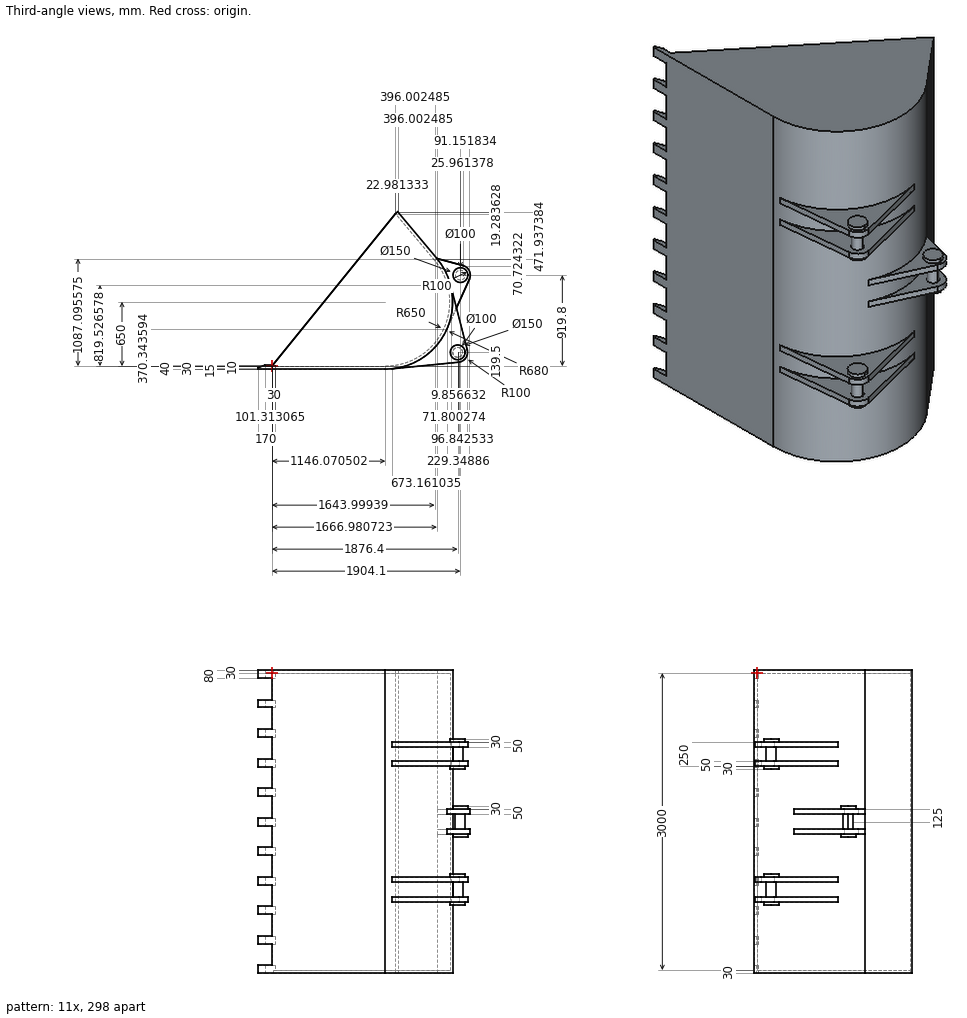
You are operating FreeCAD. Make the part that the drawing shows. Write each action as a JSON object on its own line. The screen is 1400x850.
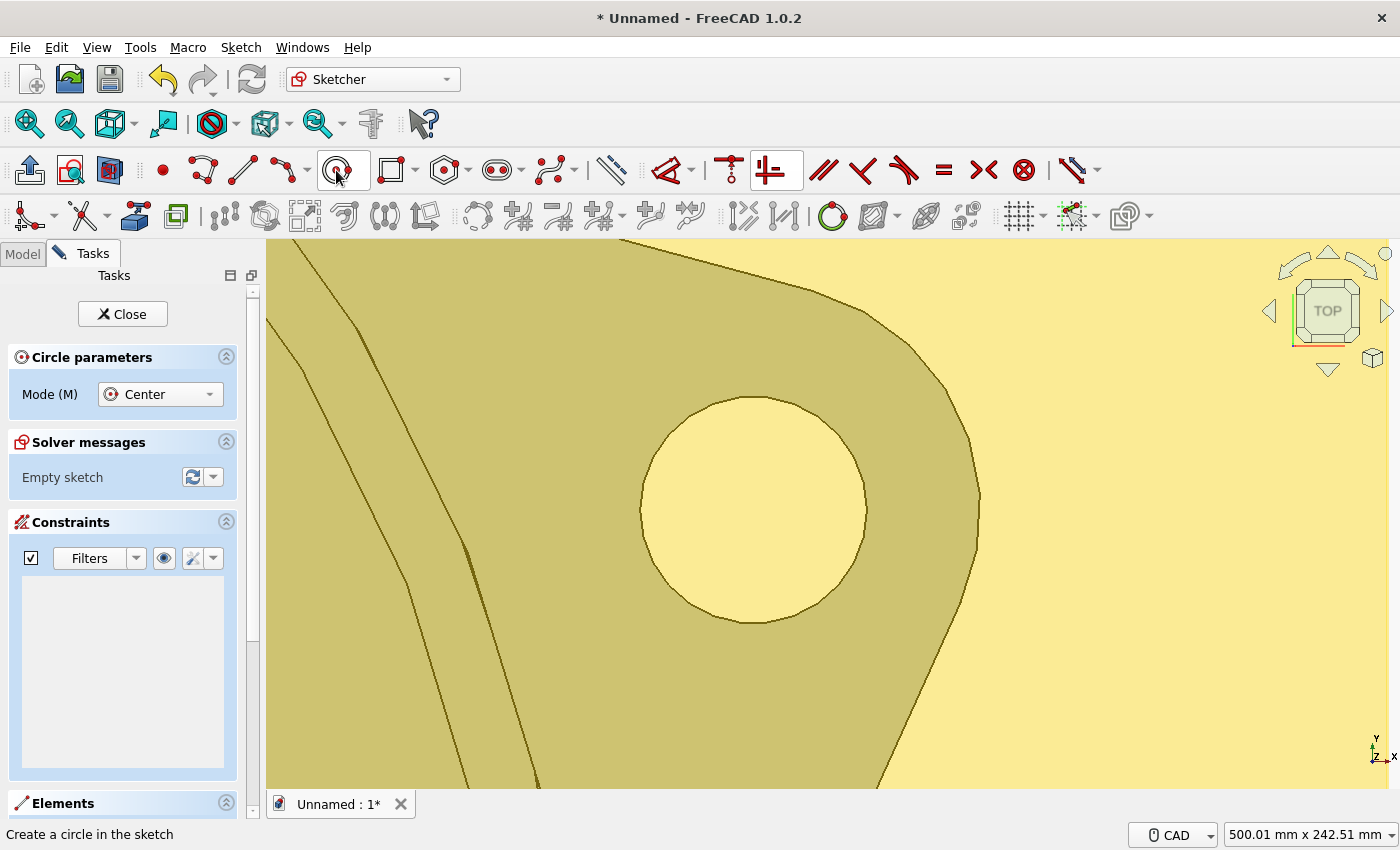
{"action": "left_click", "coordinate": [754, 510]}
{"action": "left_click", "coordinate": [874, 390]}
{"action": "key", "text": "Escape"}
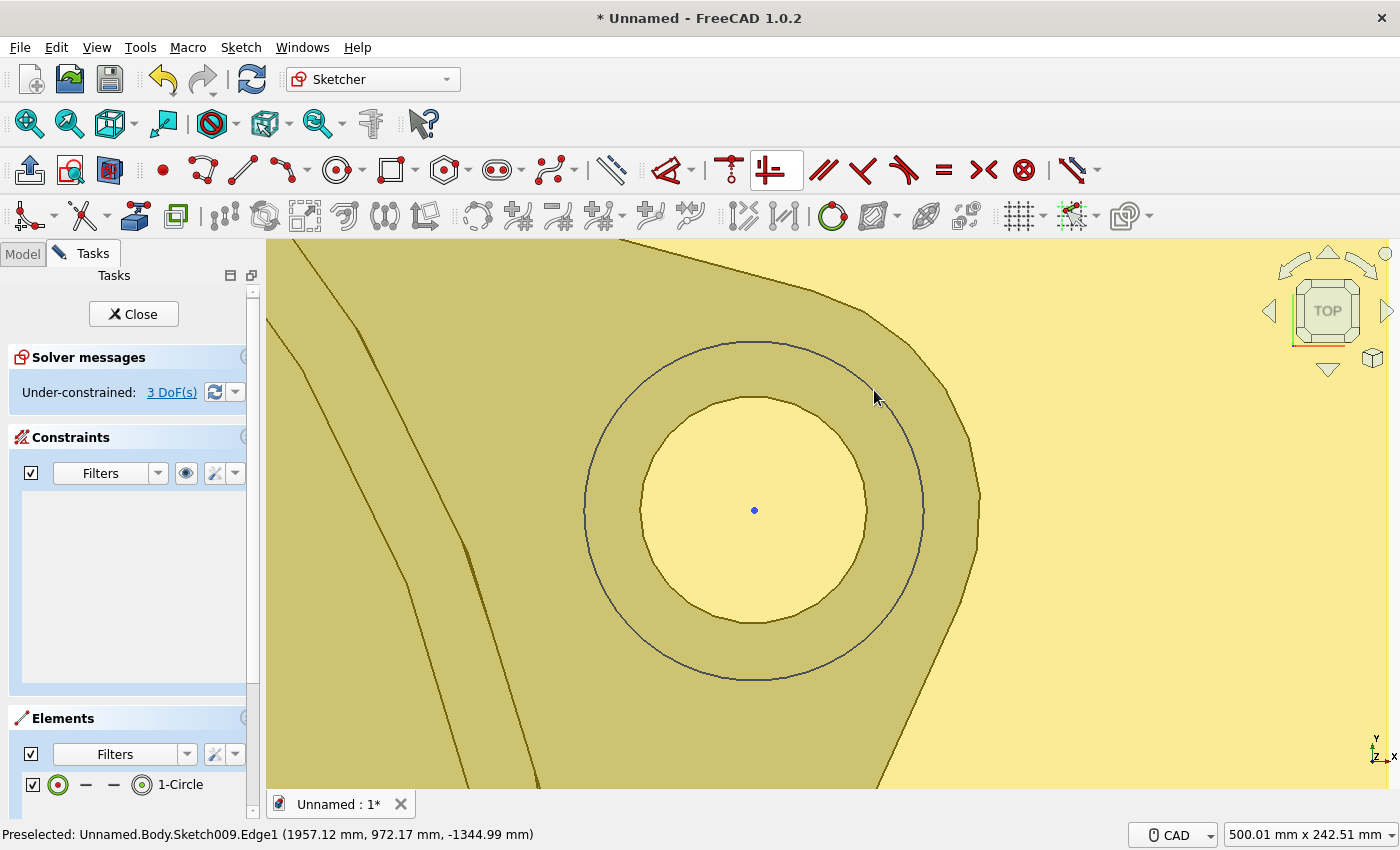
{"action": "left_click", "coordinate": [666, 170]}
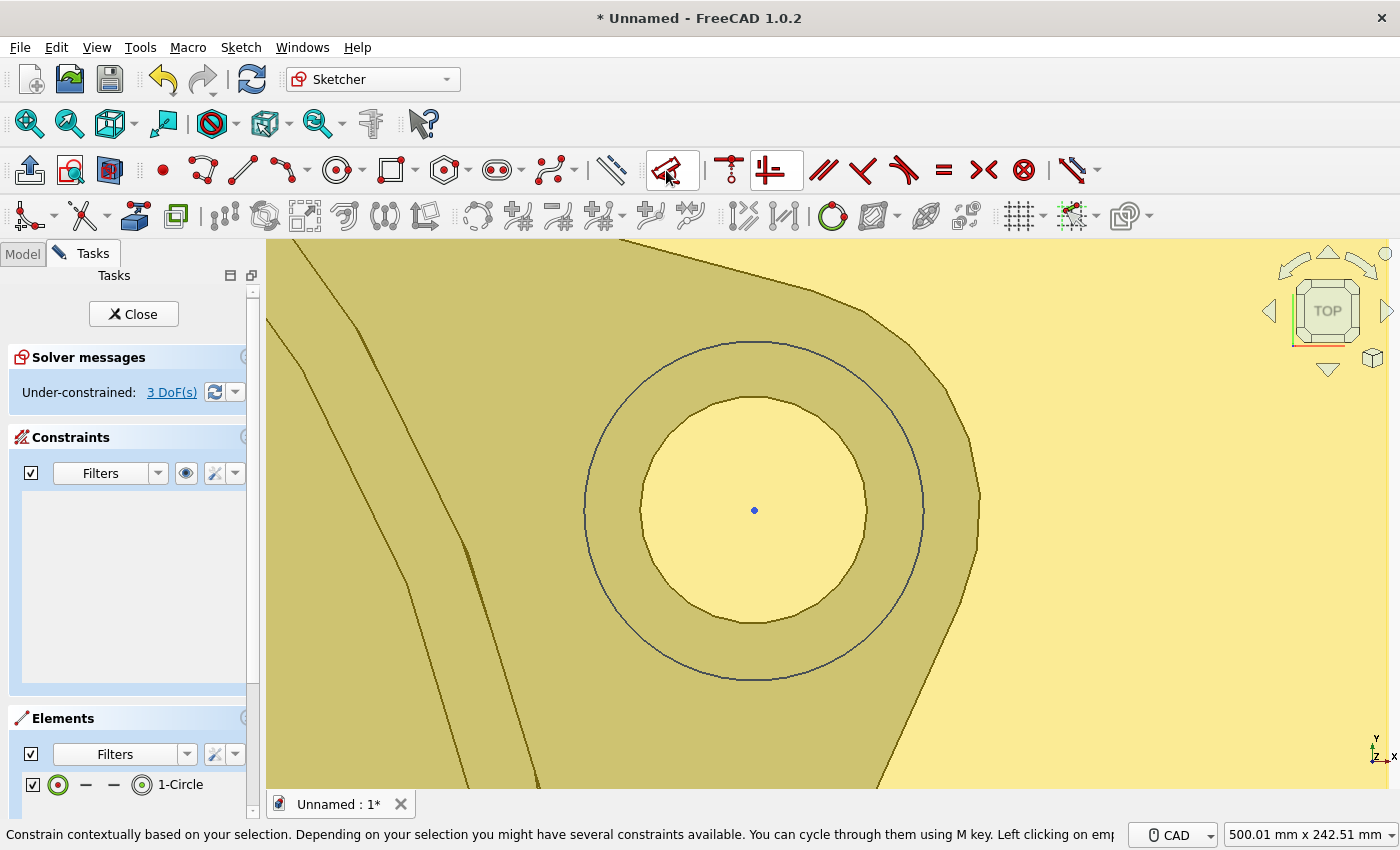
{"action": "left_click", "coordinate": [874, 391]}
{"action": "left_click", "coordinate": [897, 368]}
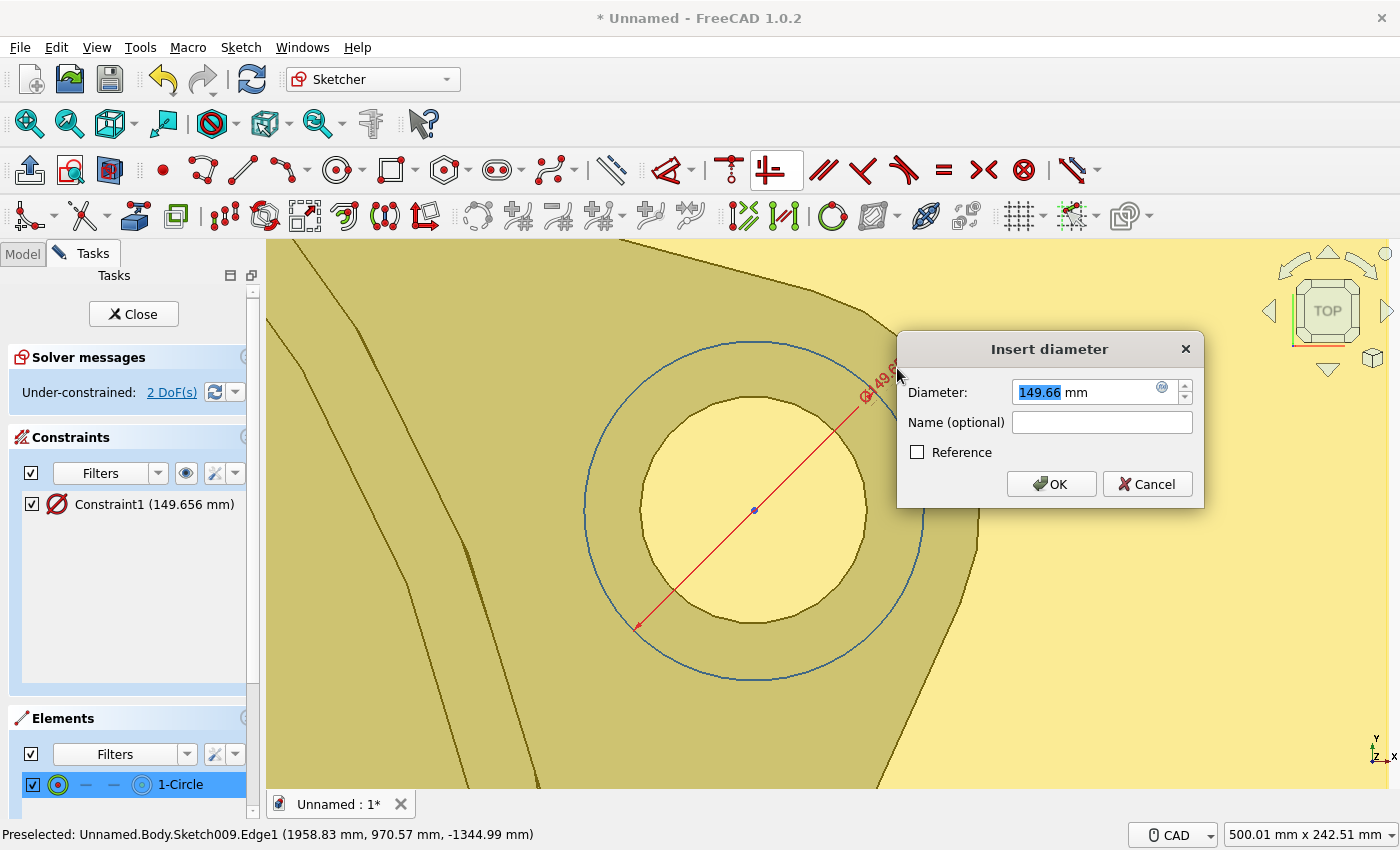
{"action": "type", "text": "150"}
{"action": "key", "text": "Return"}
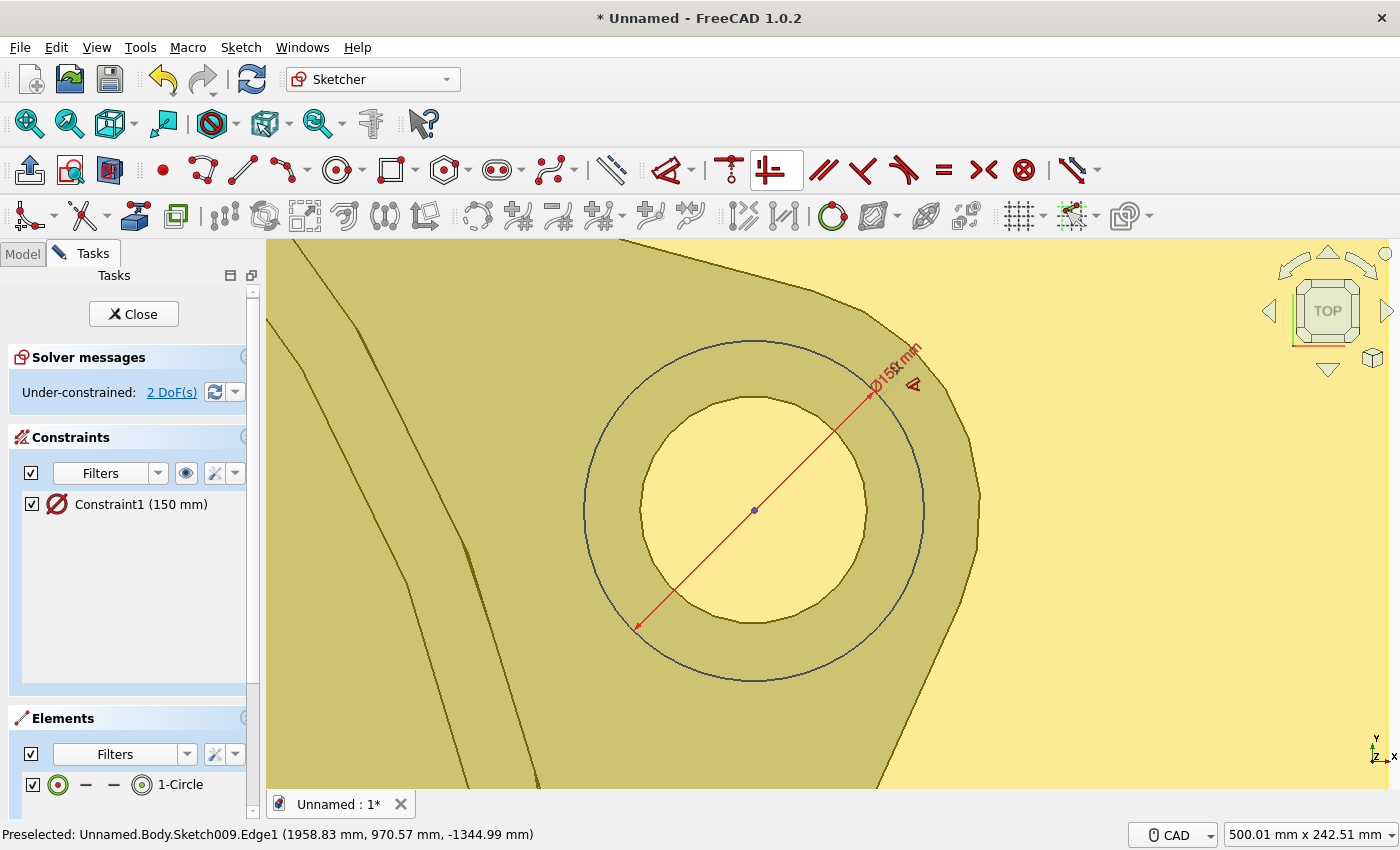
{"action": "left_click", "coordinate": [754, 511]}
{"action": "left_click", "coordinate": [788, 636]}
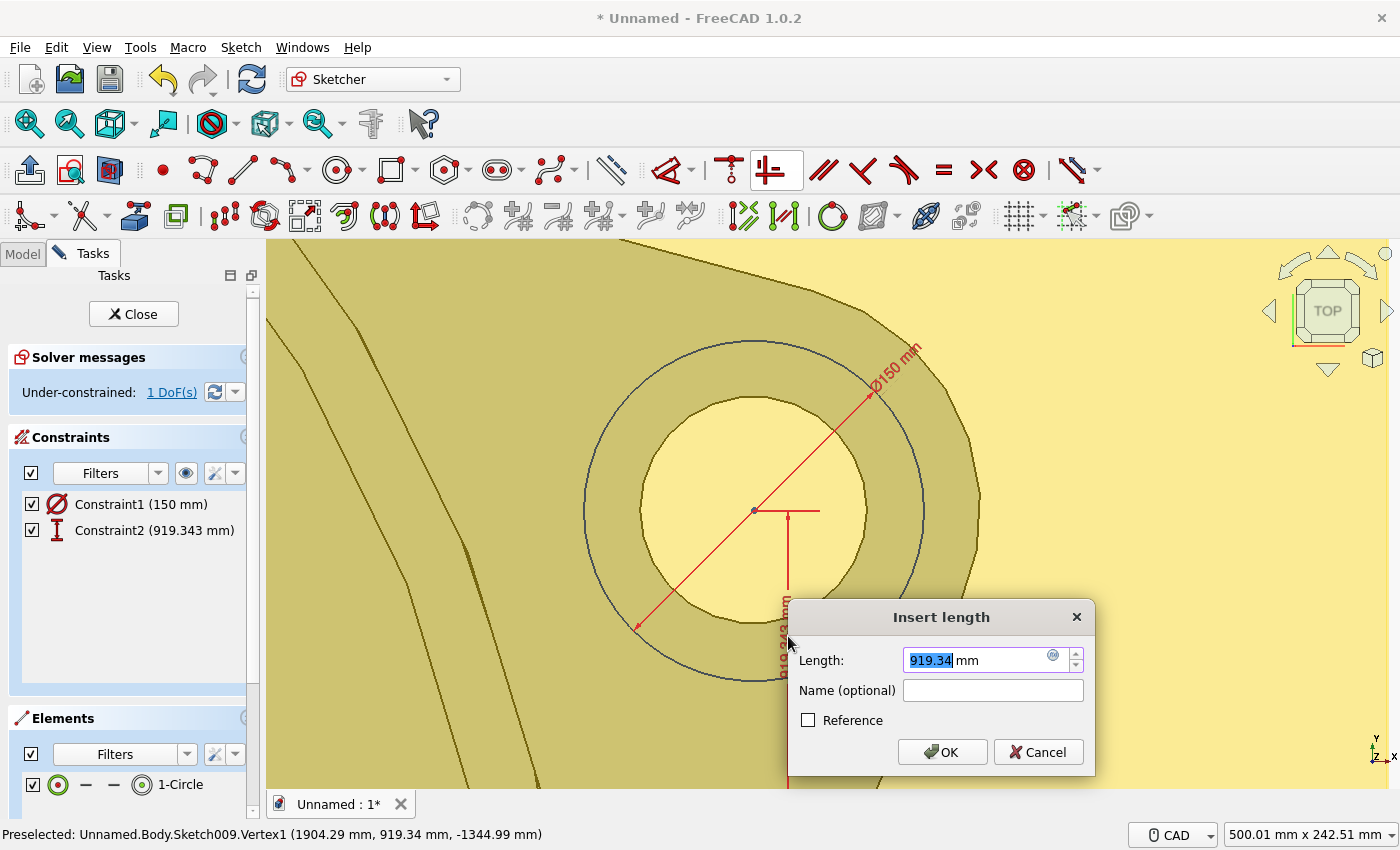
{"action": "type", "text": "919.8"}
{"action": "key", "text": "Return"}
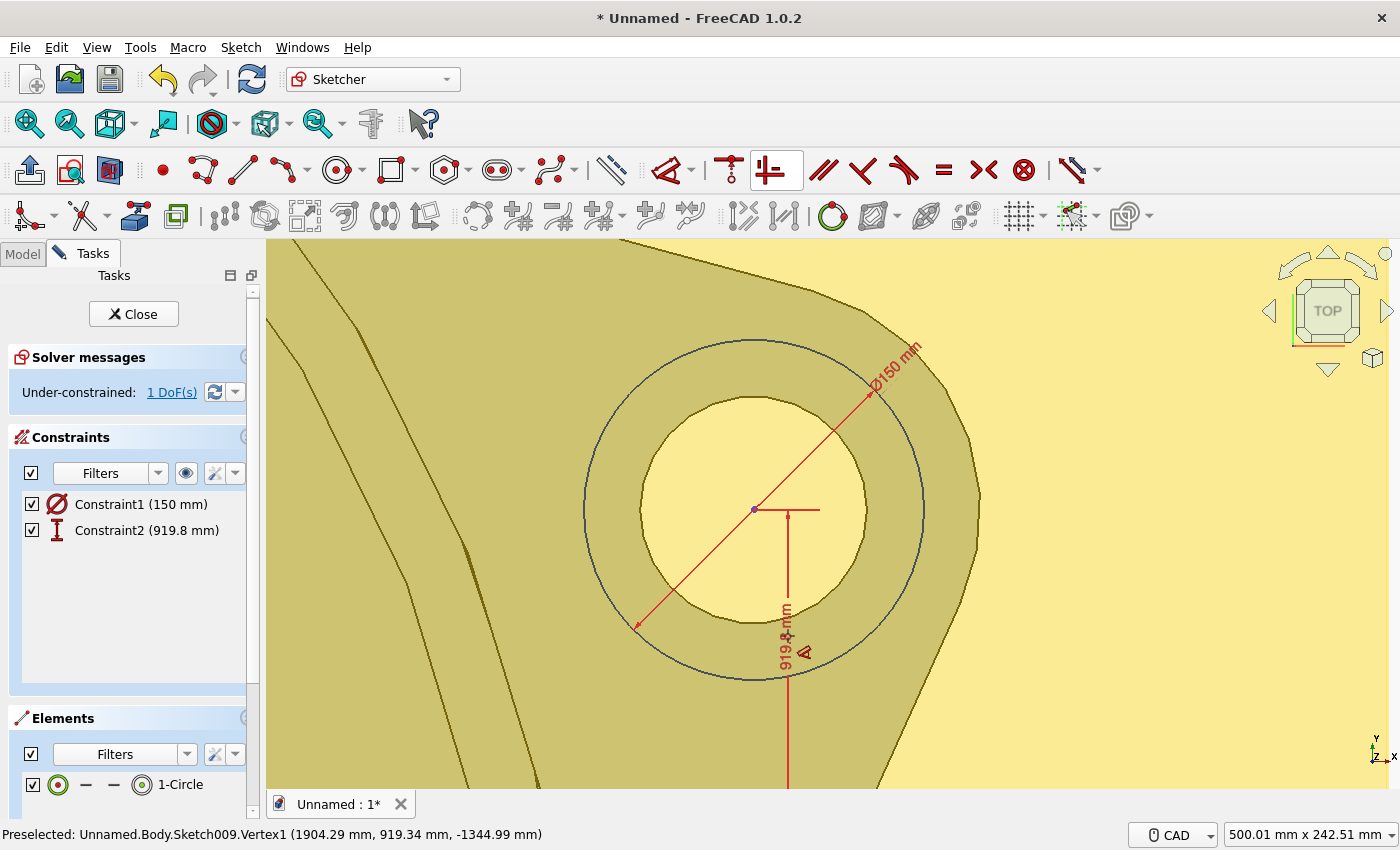
{"action": "left_click", "coordinate": [754, 510]}
{"action": "left_click", "coordinate": [524, 476]}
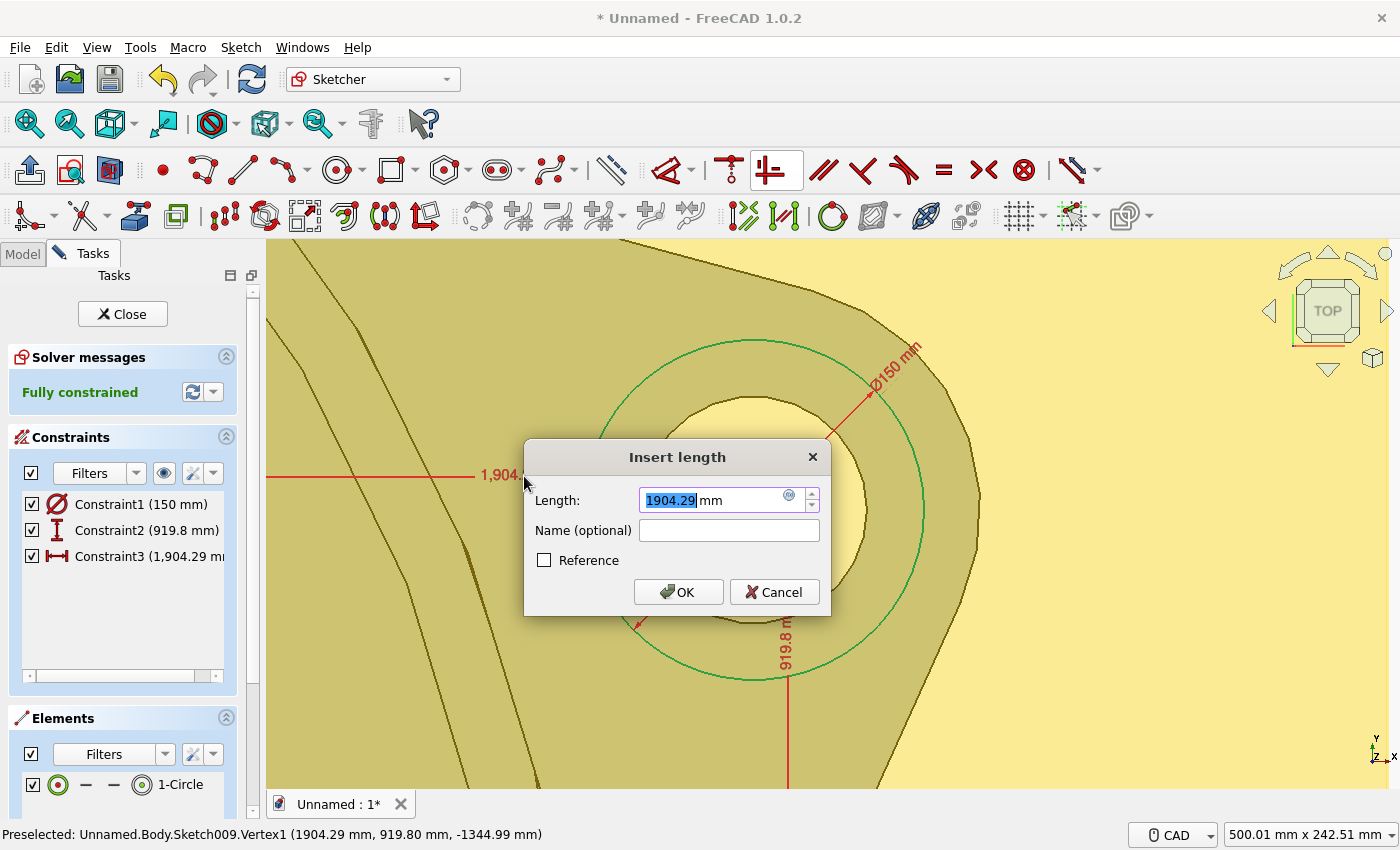
{"action": "type", "text": "1904.1"}
{"action": "key", "text": "Return"}
{"action": "key", "text": "Escape"}